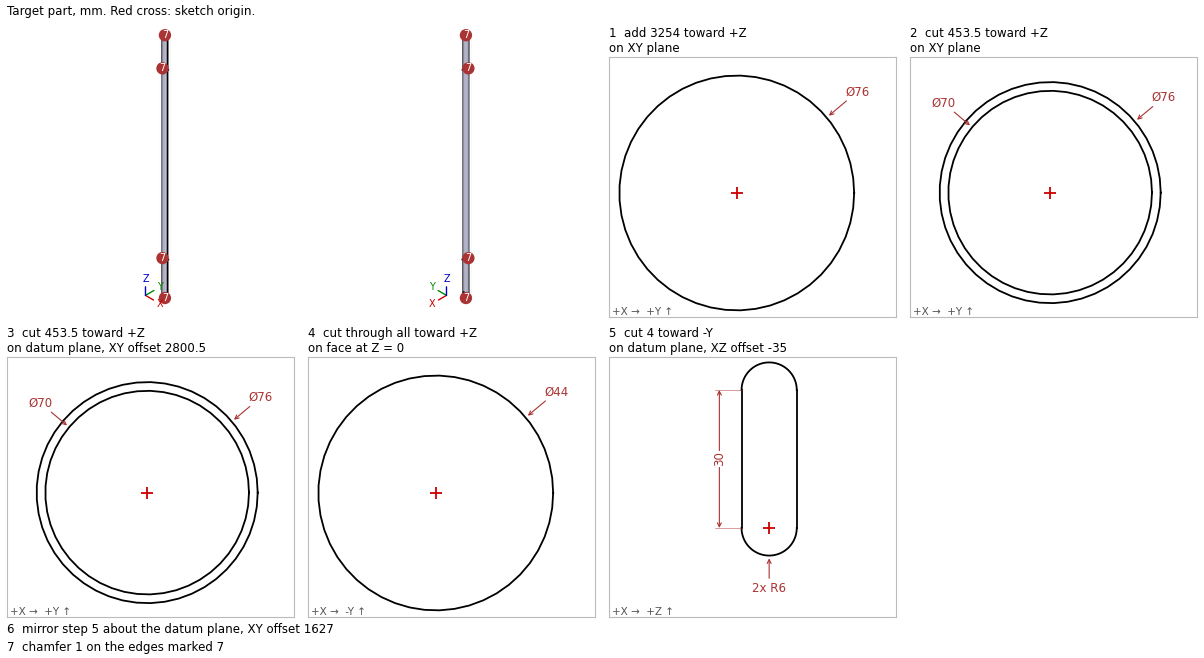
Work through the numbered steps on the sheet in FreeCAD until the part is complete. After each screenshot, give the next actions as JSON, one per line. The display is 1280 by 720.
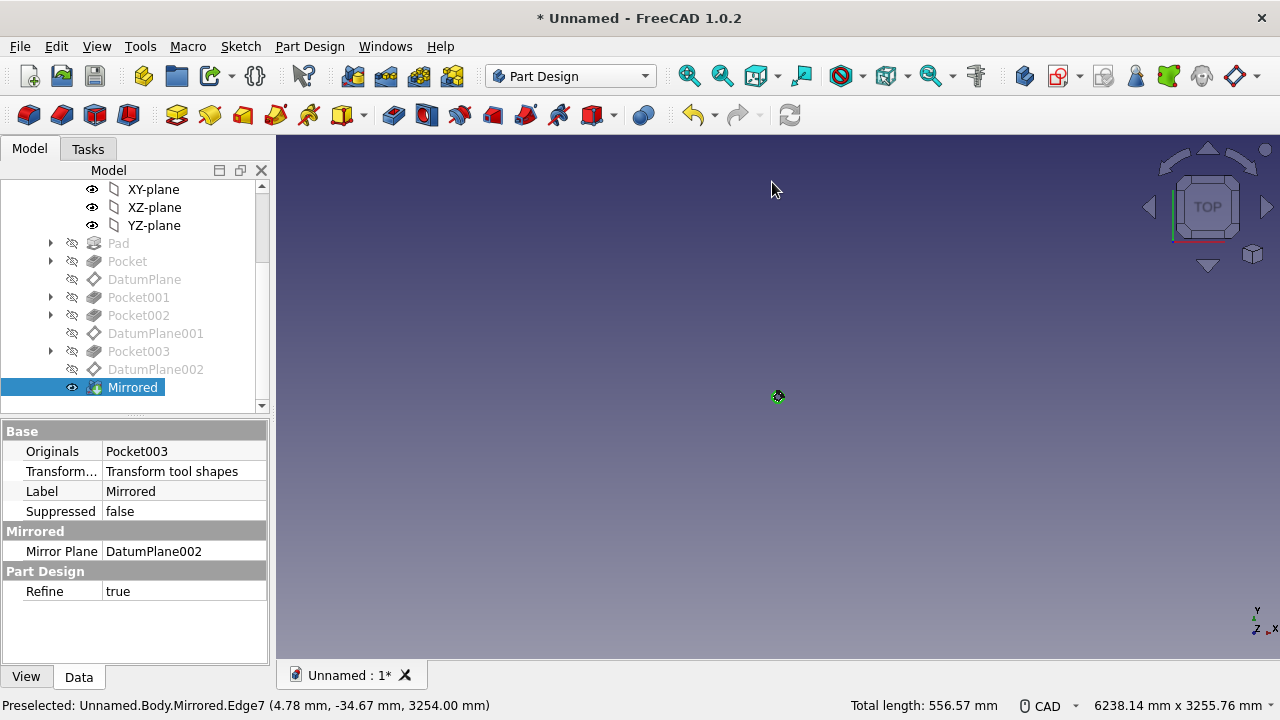
{"action": "left_click", "coordinate": [690, 76]}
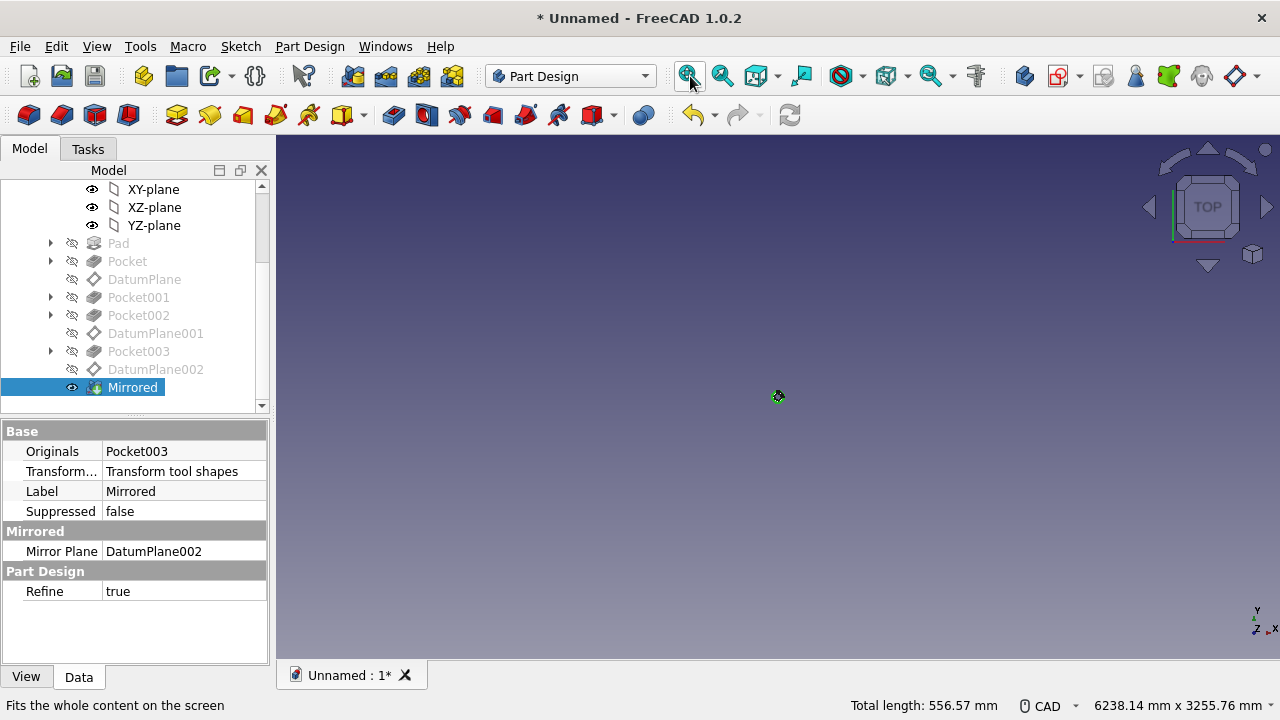
{"action": "key", "text": "1"}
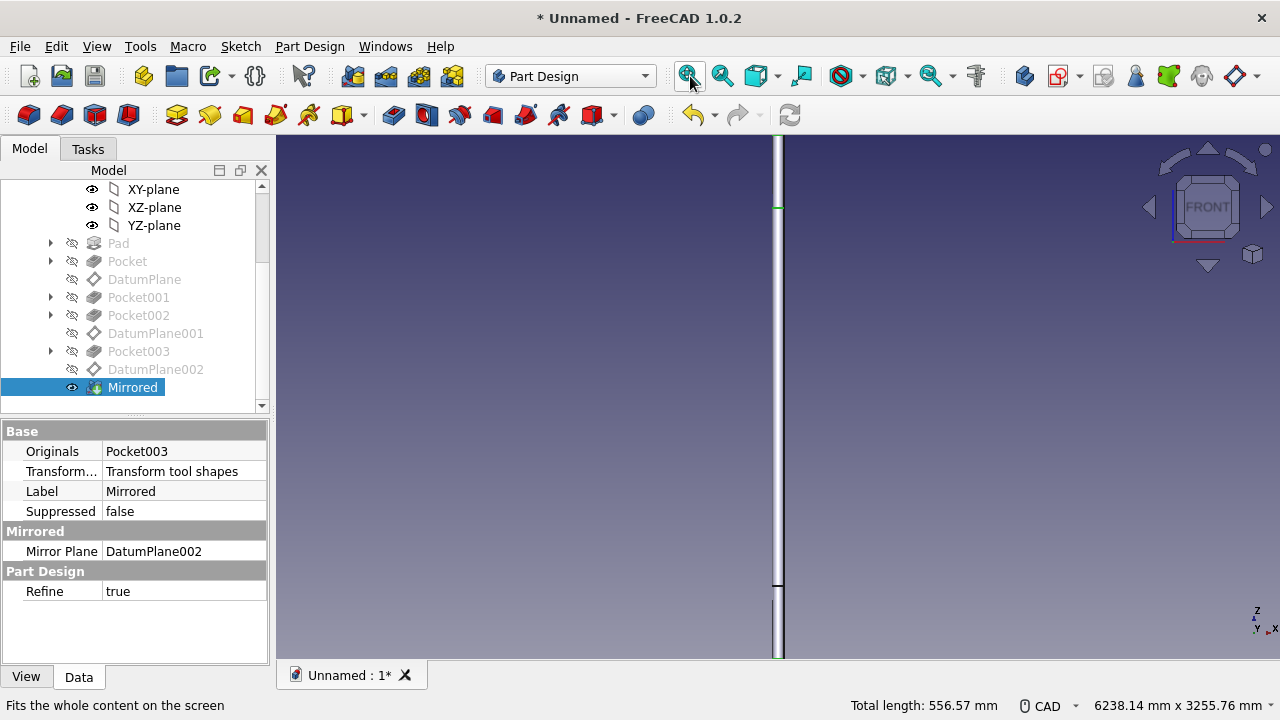
{"action": "left_click", "coordinate": [690, 76]}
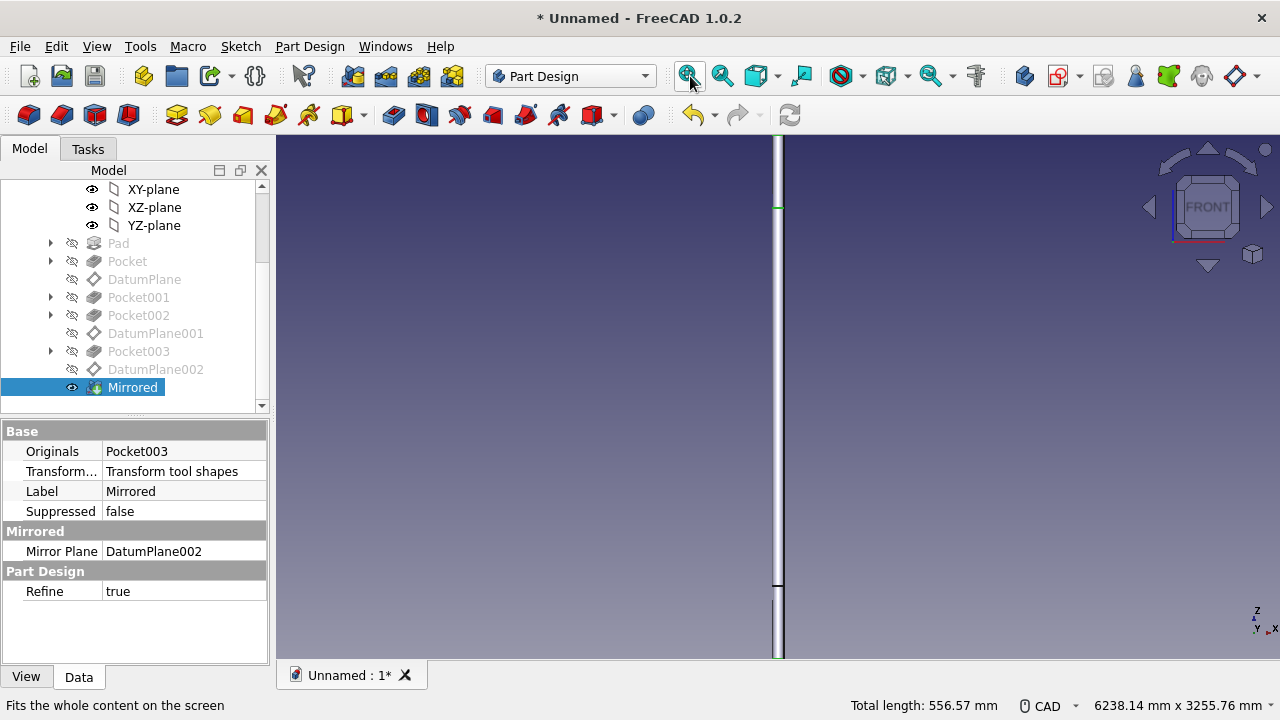
{"action": "left_click", "coordinate": [772, 585], "text": "ctrl"}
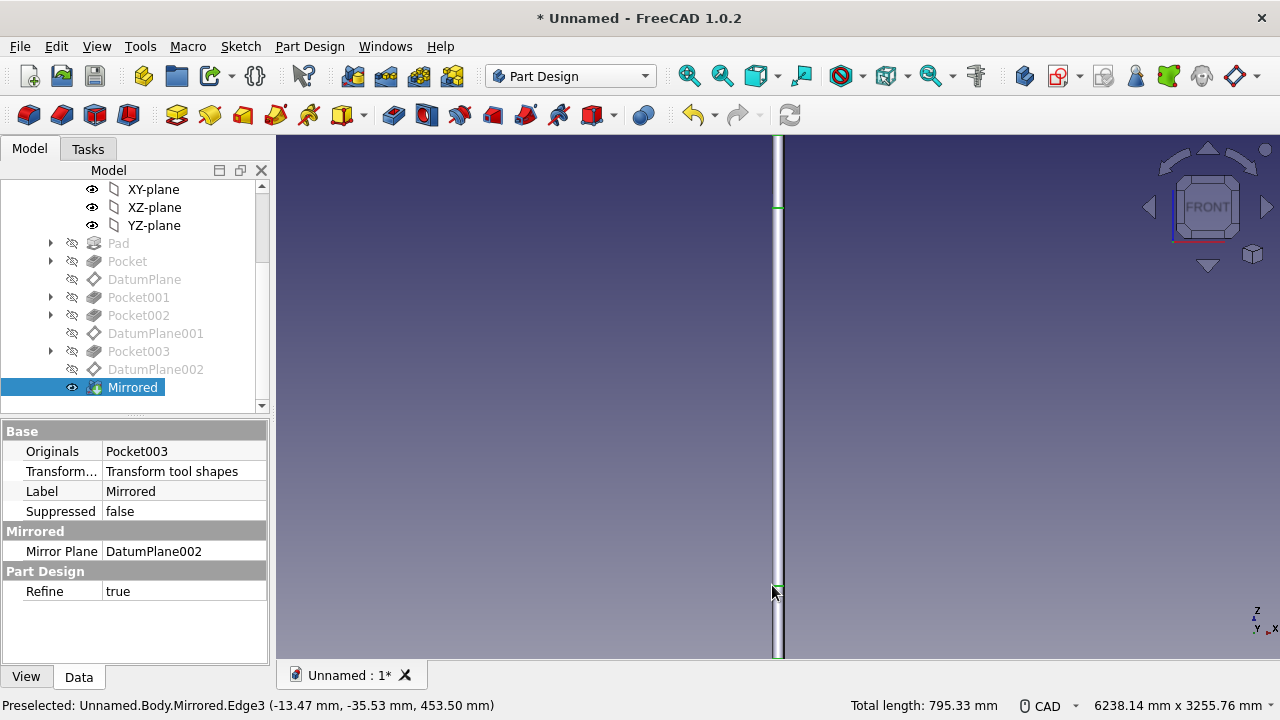
{"action": "left_click", "coordinate": [62, 116]}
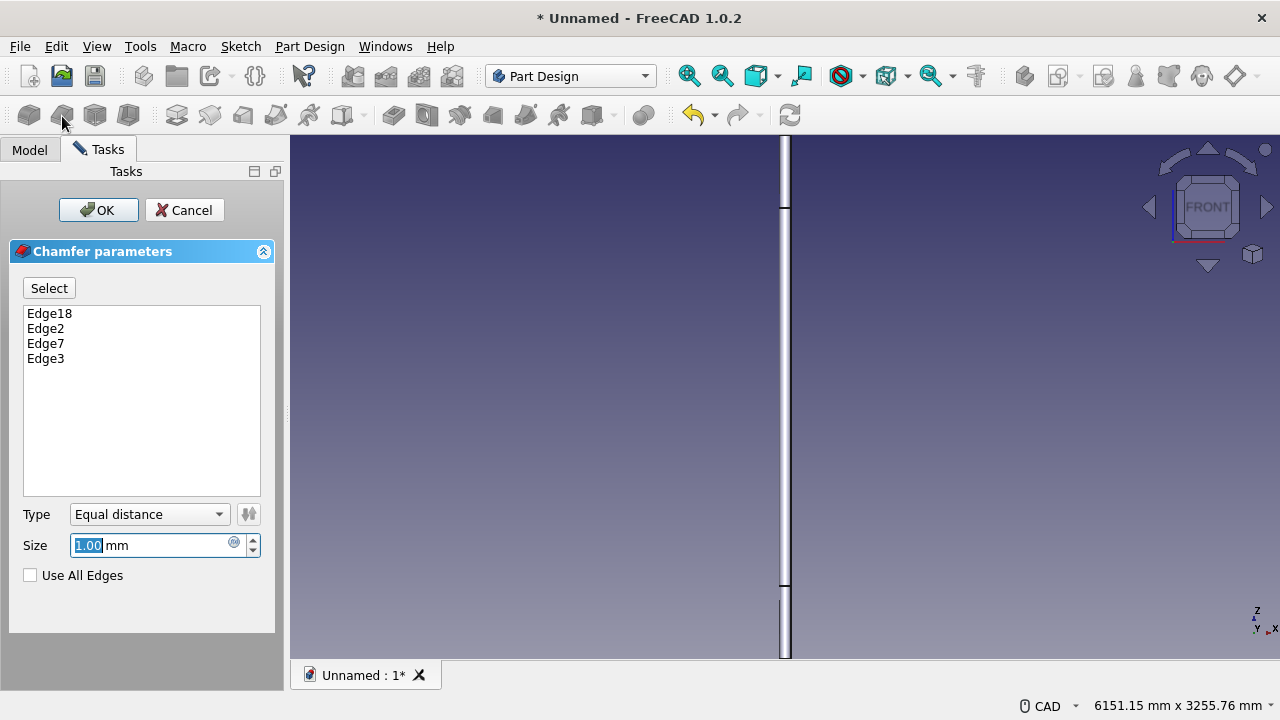
{"action": "type", "text": "1"}
{"action": "key", "text": "Tab"}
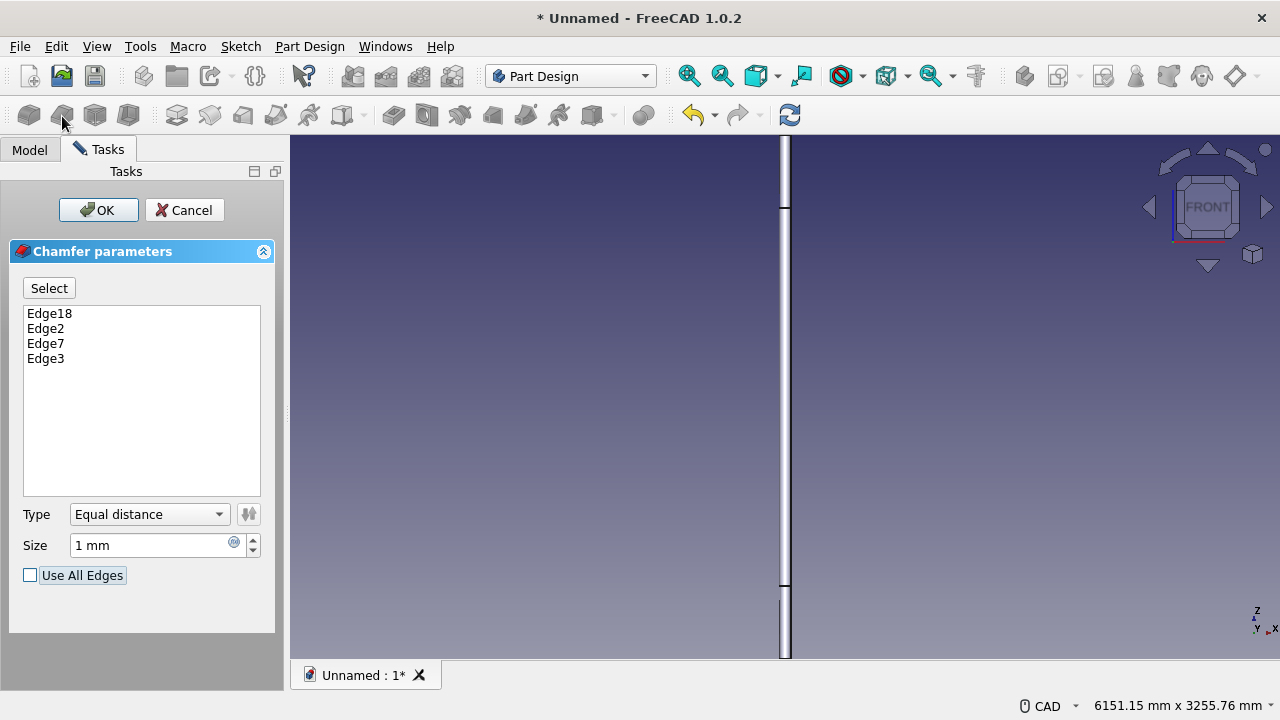
{"action": "left_click", "coordinate": [99, 210]}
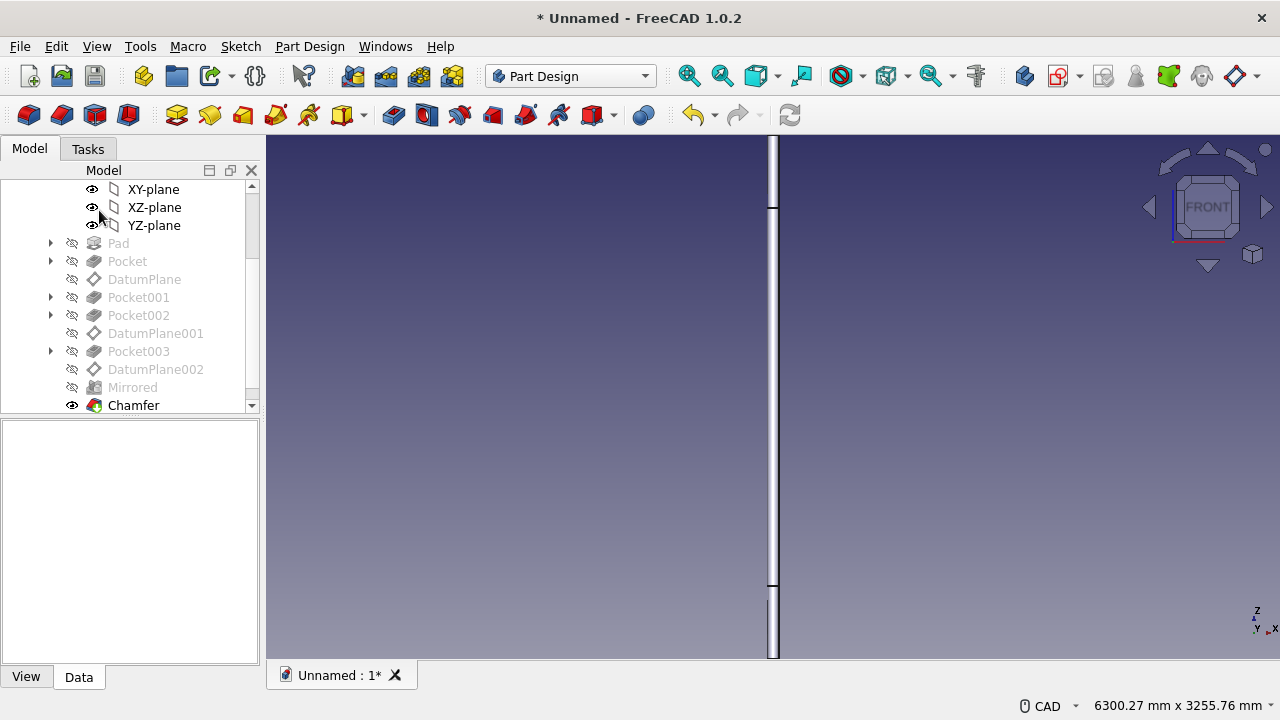
{"action": "key", "text": "0"}